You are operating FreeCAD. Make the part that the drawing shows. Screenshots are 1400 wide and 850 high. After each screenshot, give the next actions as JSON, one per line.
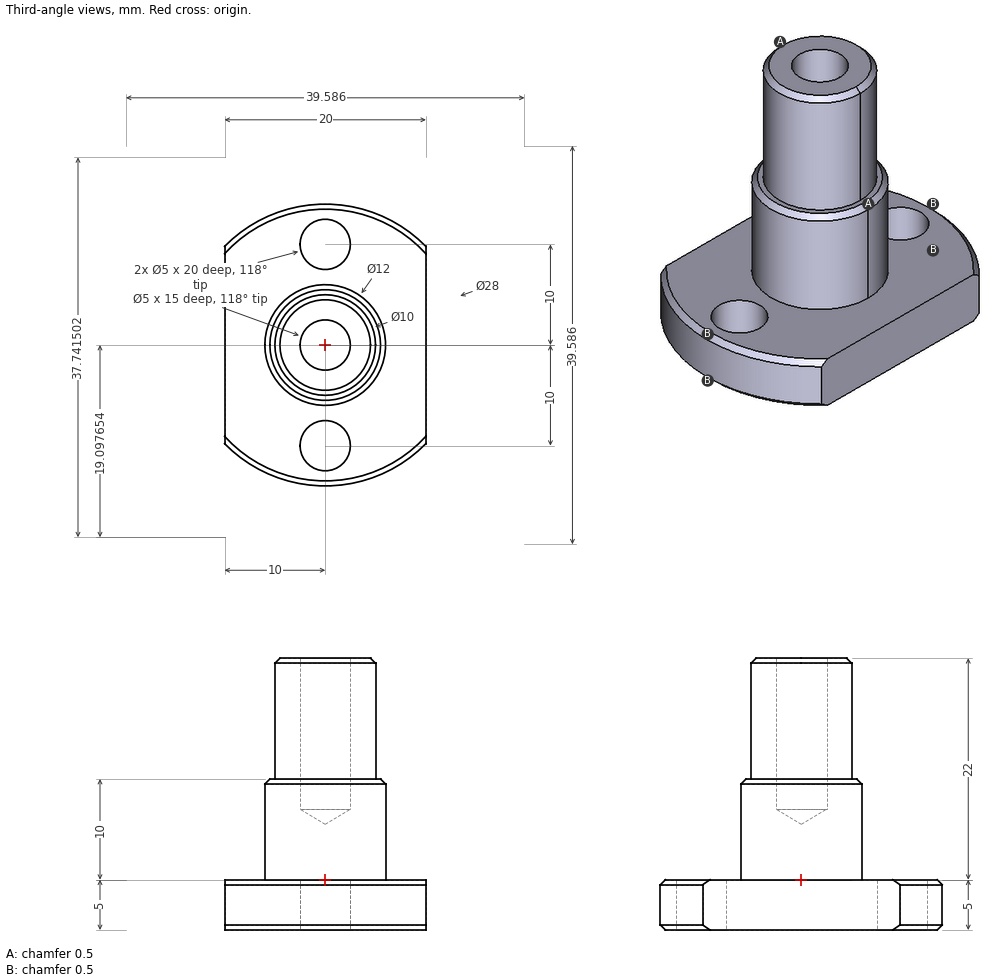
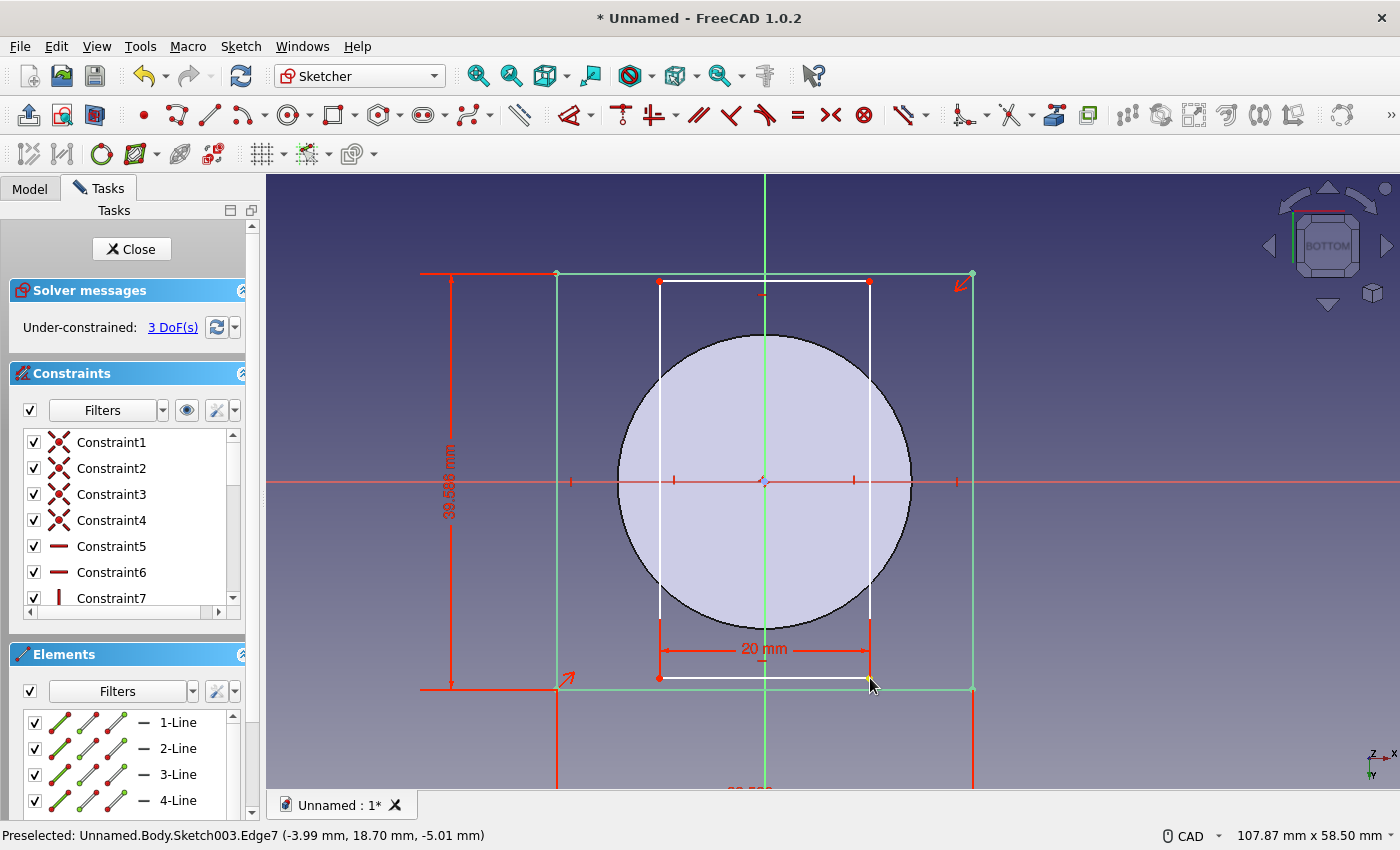
{"action": "left_click", "coordinate": [660, 281]}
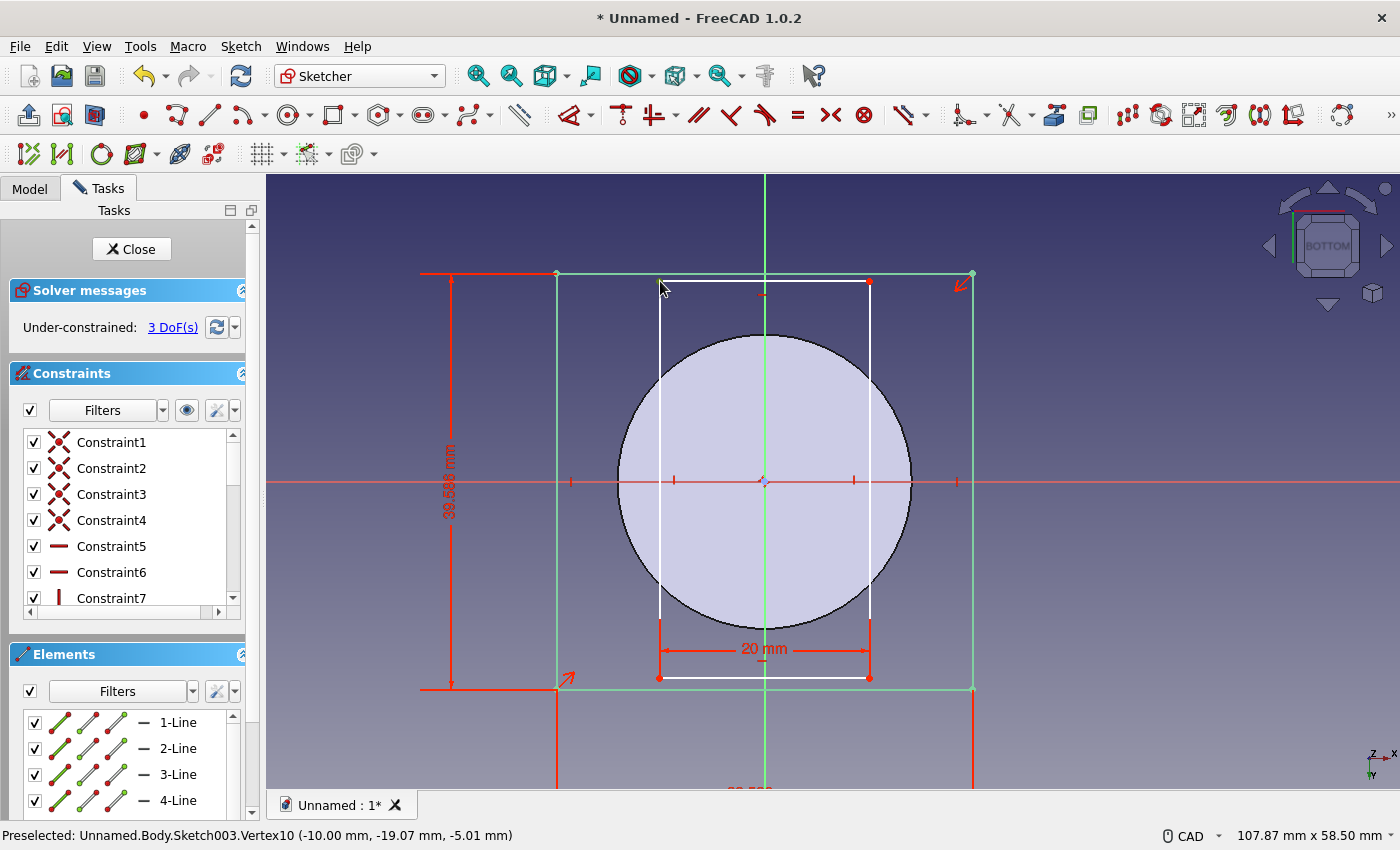
{"action": "key", "text": "l"}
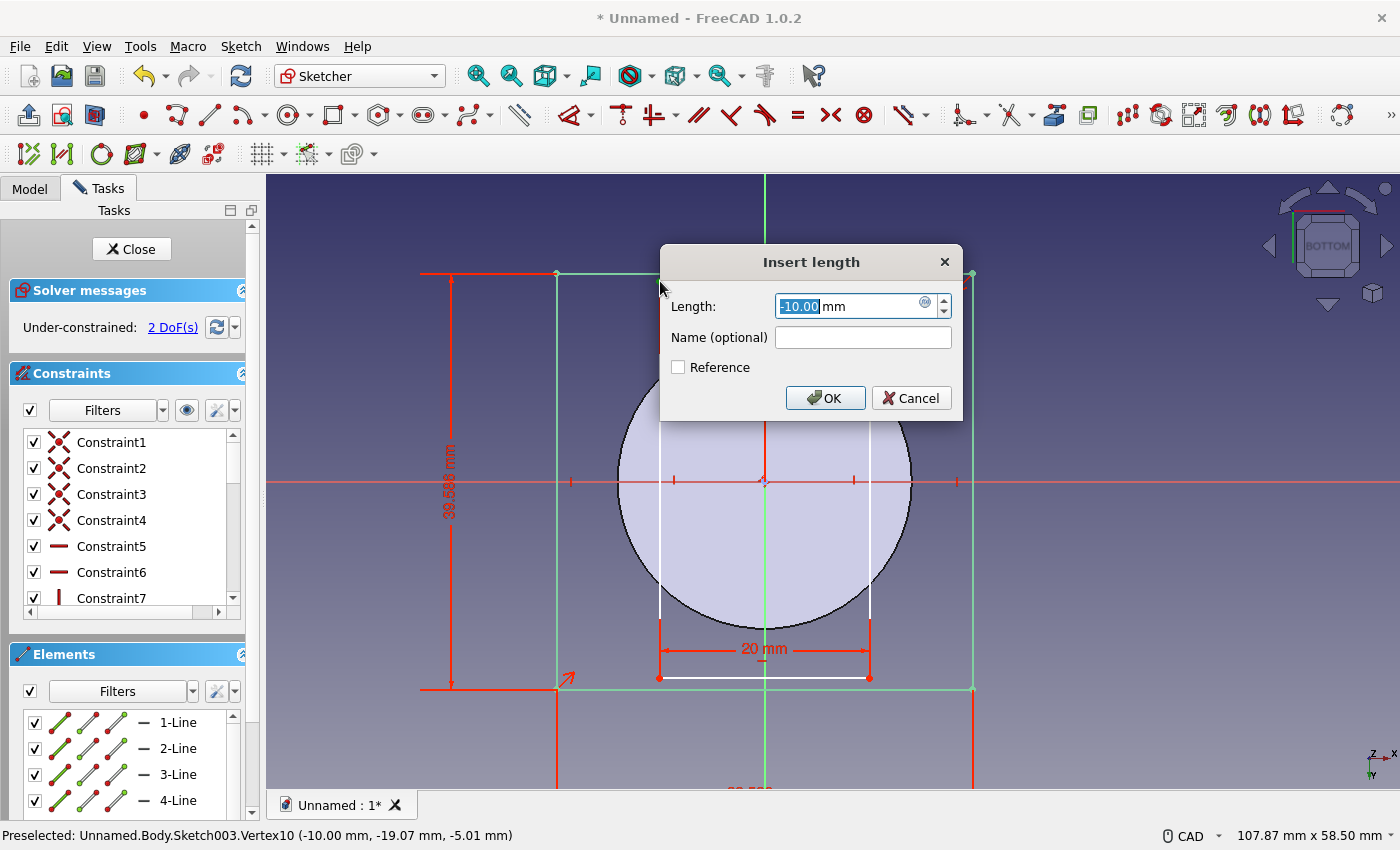
{"action": "type", "text": "-10"}
{"action": "key", "text": "Return"}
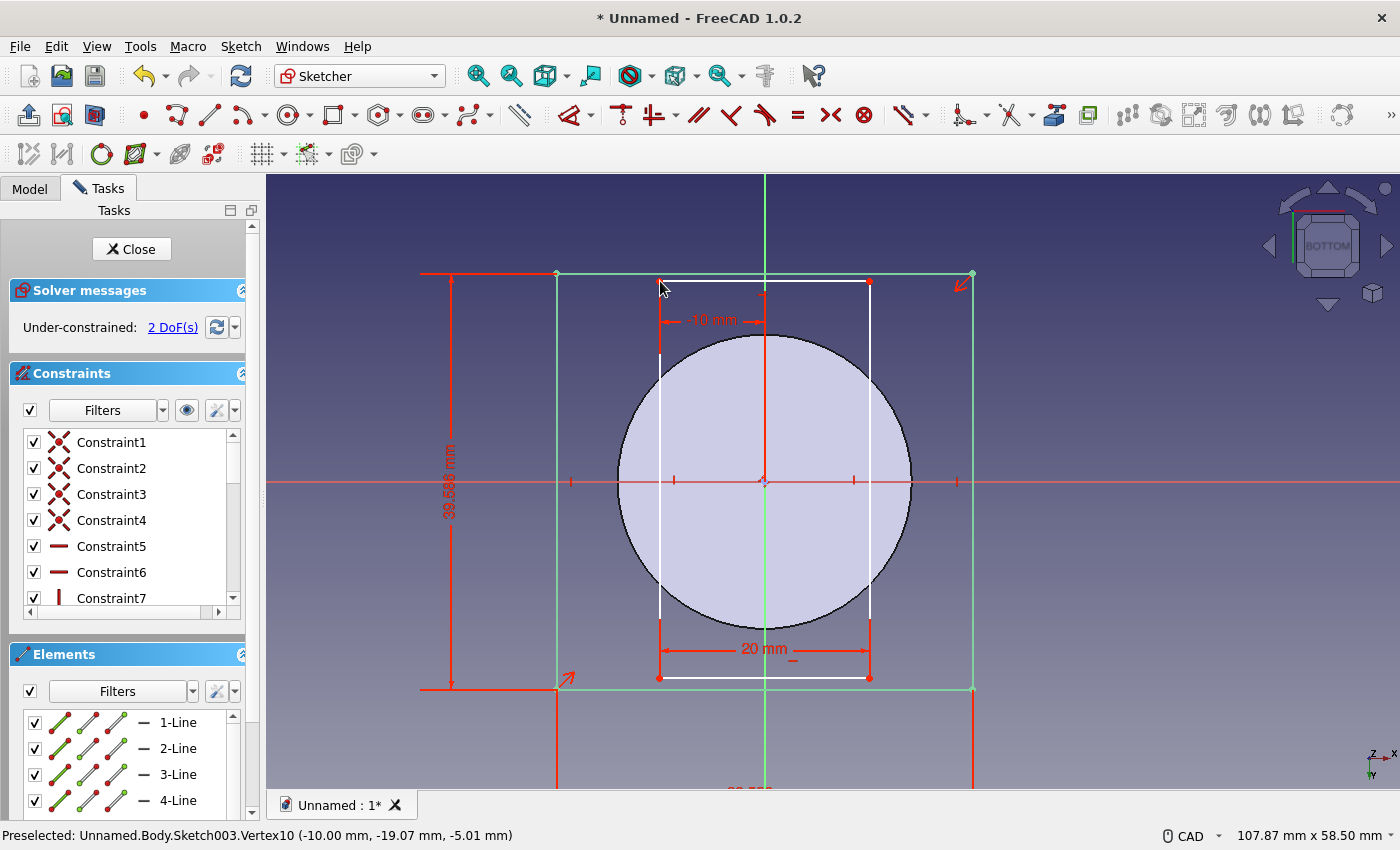
{"action": "left_click", "coordinate": [660, 400]}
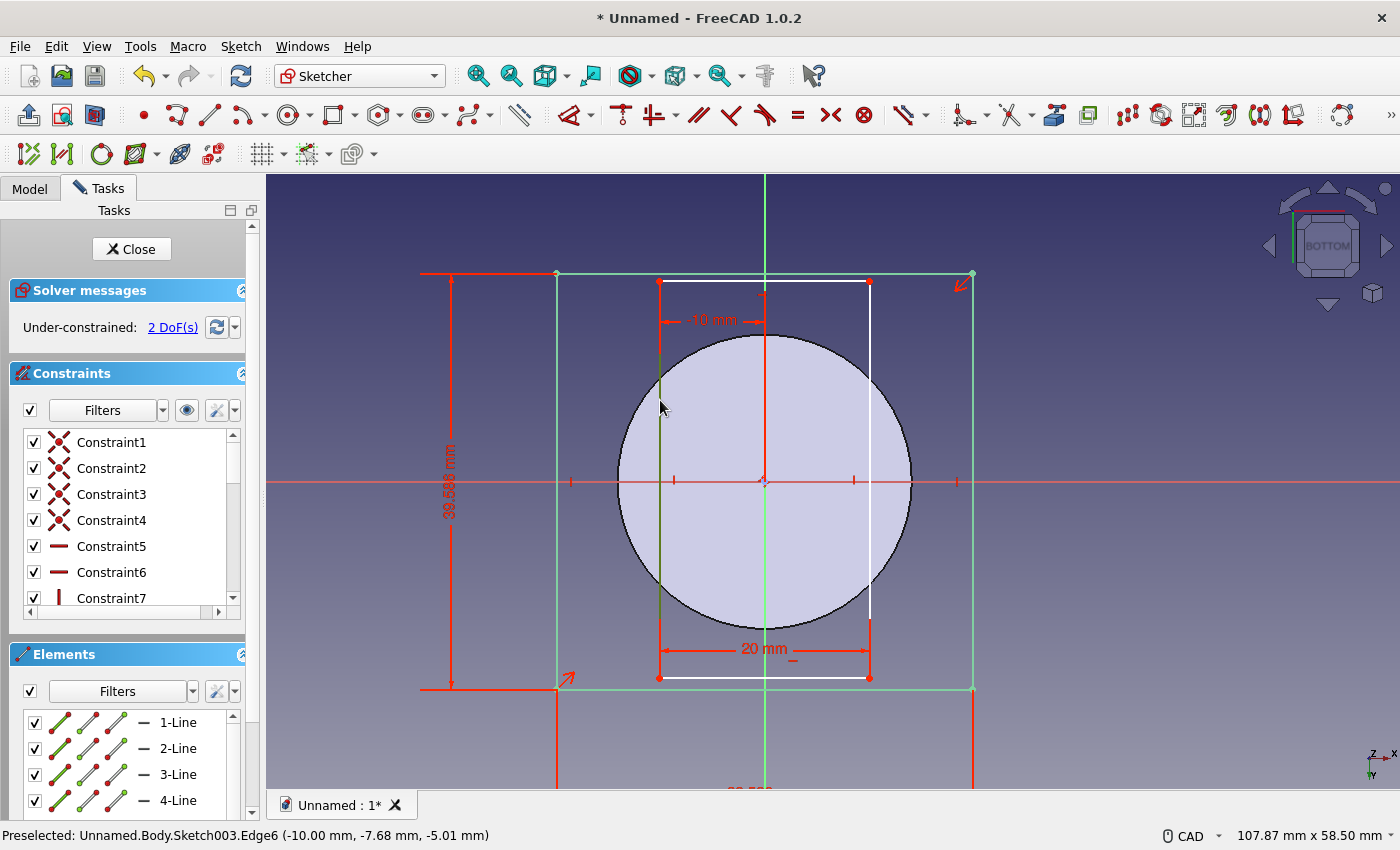
{"action": "key", "text": "i"}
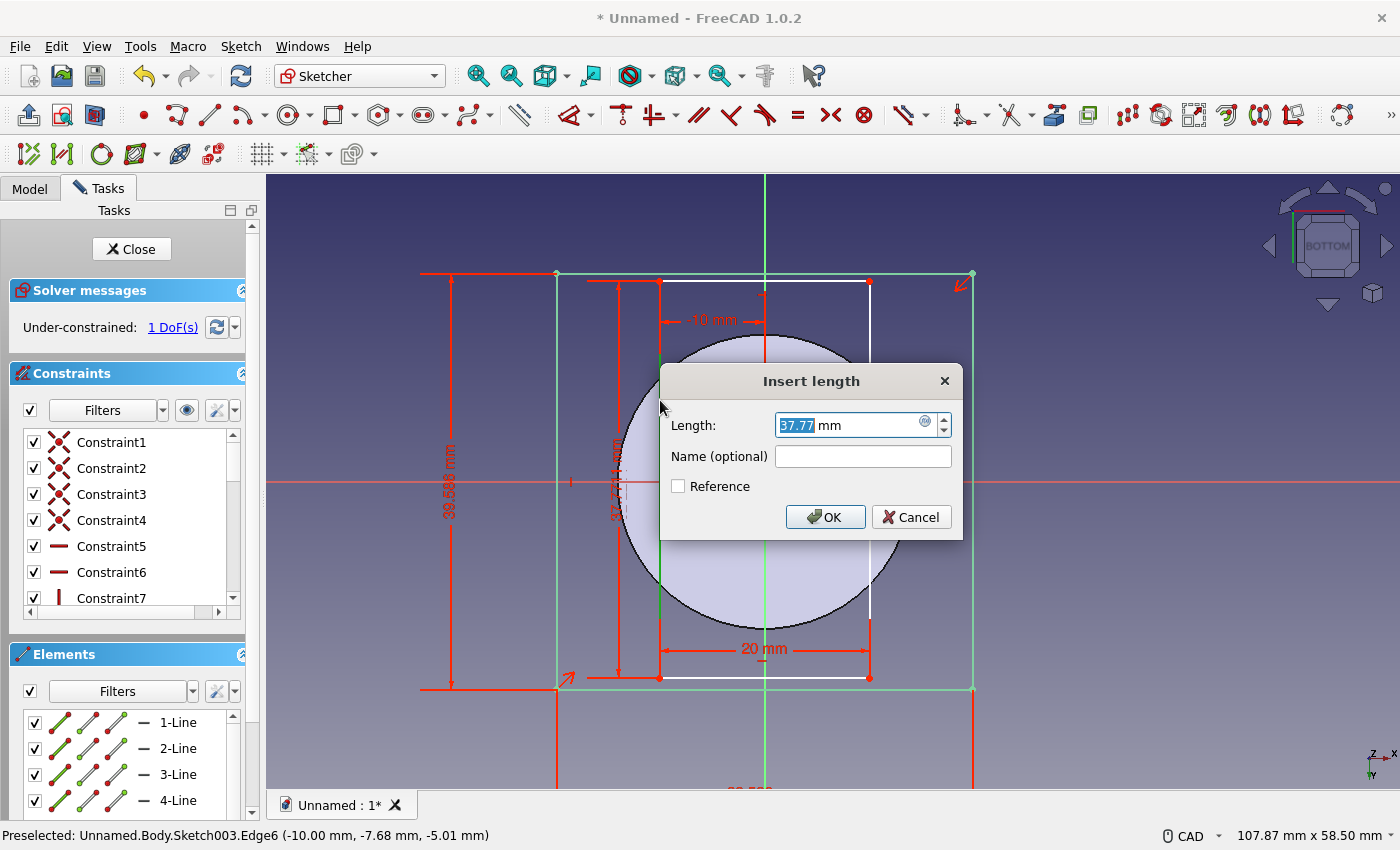
{"action": "type", "text": "37.741502"}
{"action": "key", "text": "Return"}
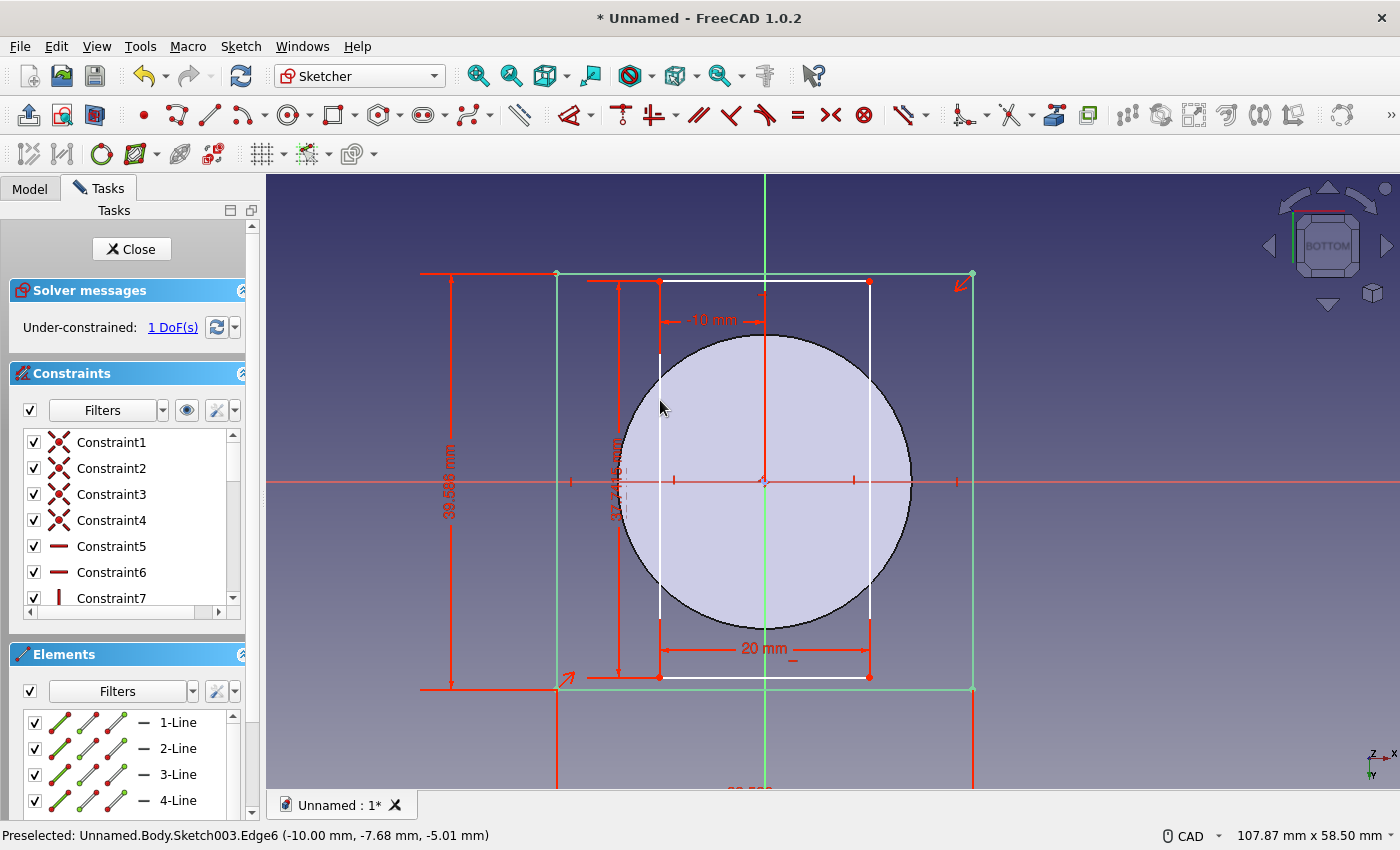
{"action": "left_click", "coordinate": [660, 281]}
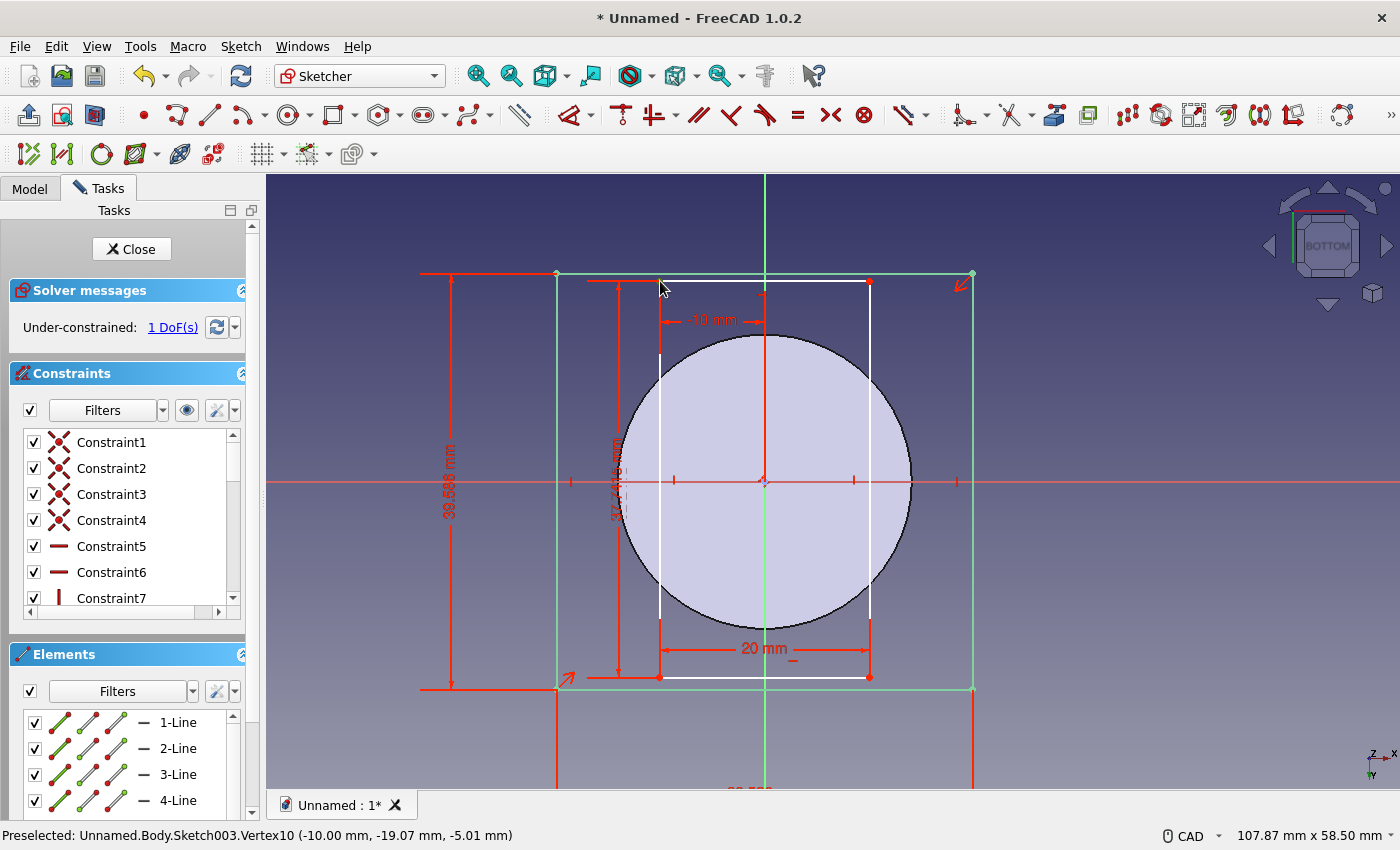
{"action": "left_click", "coordinate": [590, 116]}